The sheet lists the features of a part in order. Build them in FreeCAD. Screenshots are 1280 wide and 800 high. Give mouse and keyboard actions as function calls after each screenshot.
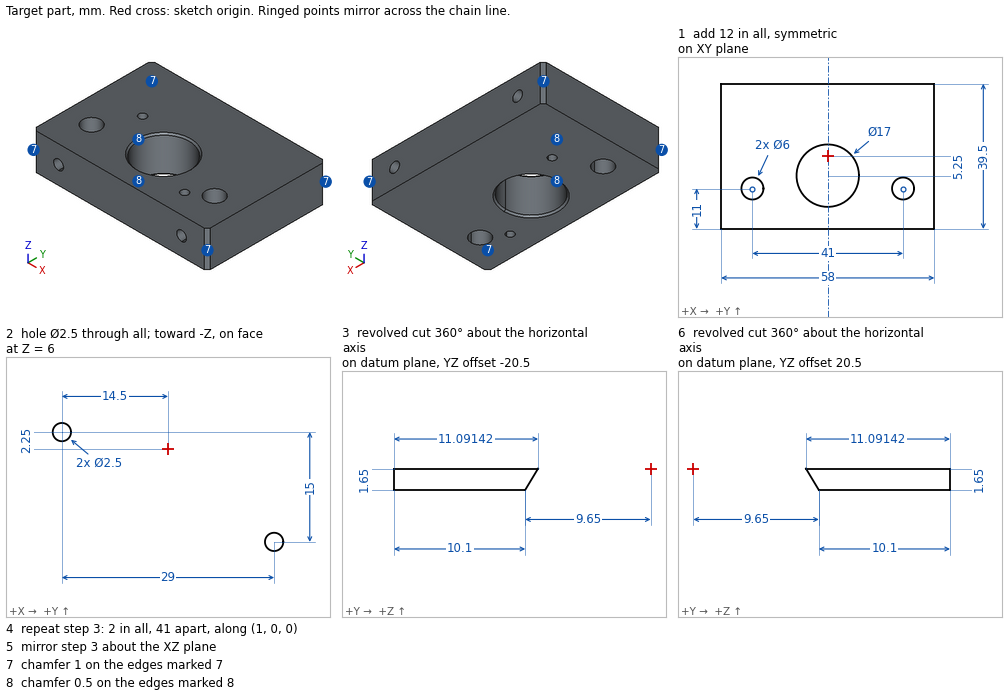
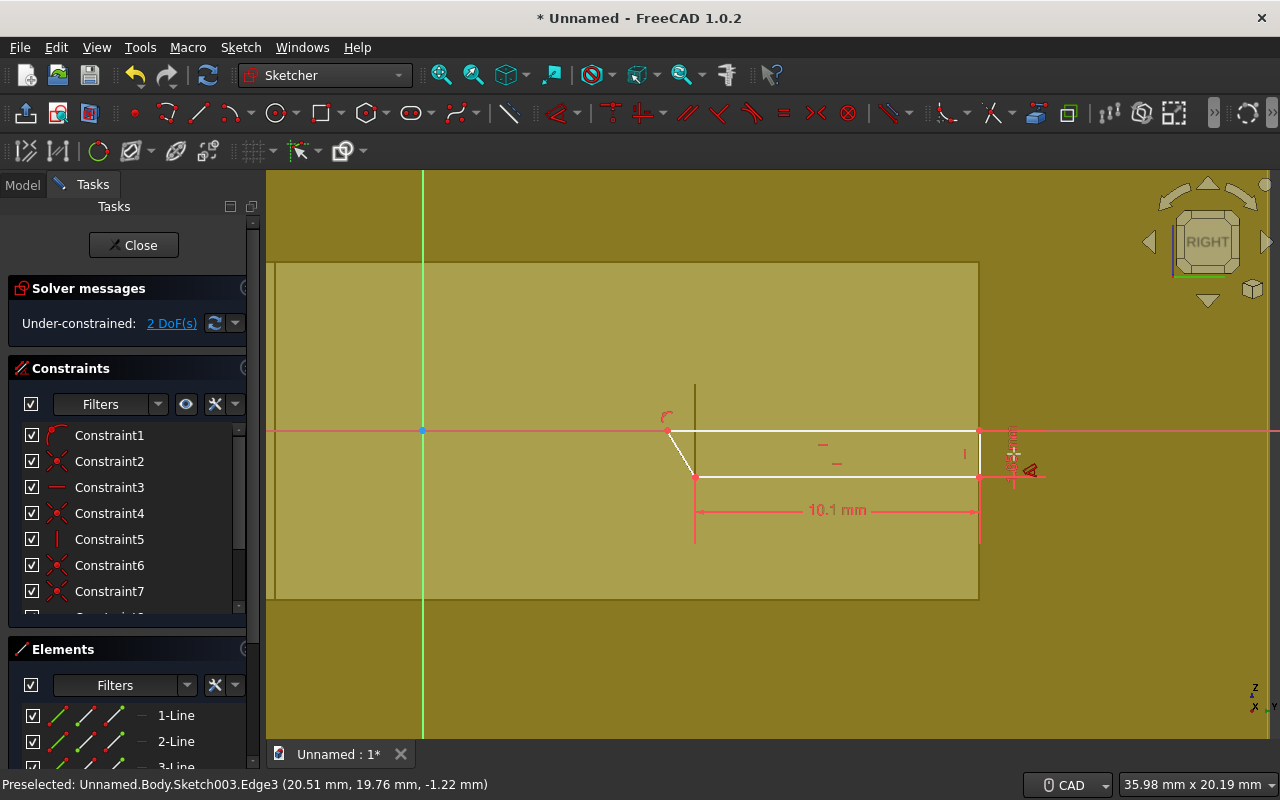
click(695, 477)
click(559, 511)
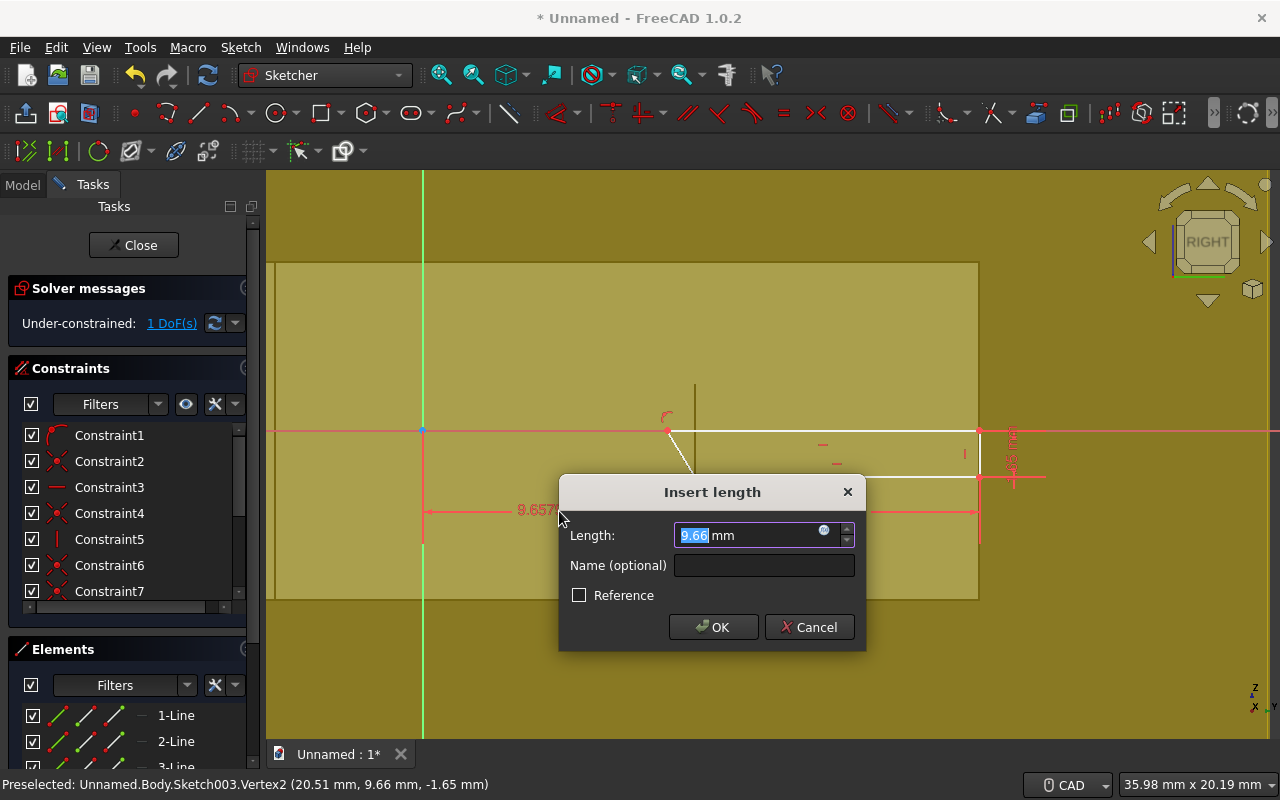
text(9.65)
key(Return)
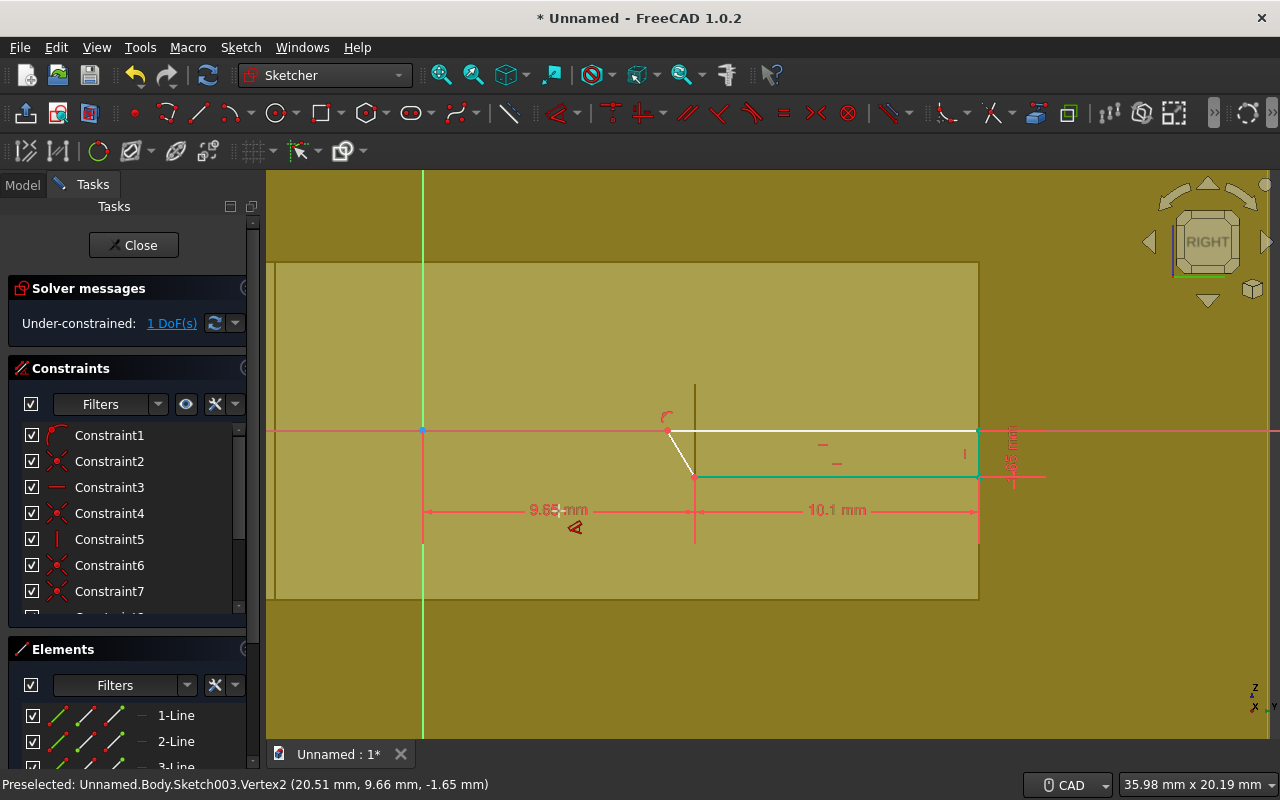
click(886, 431)
click(823, 397)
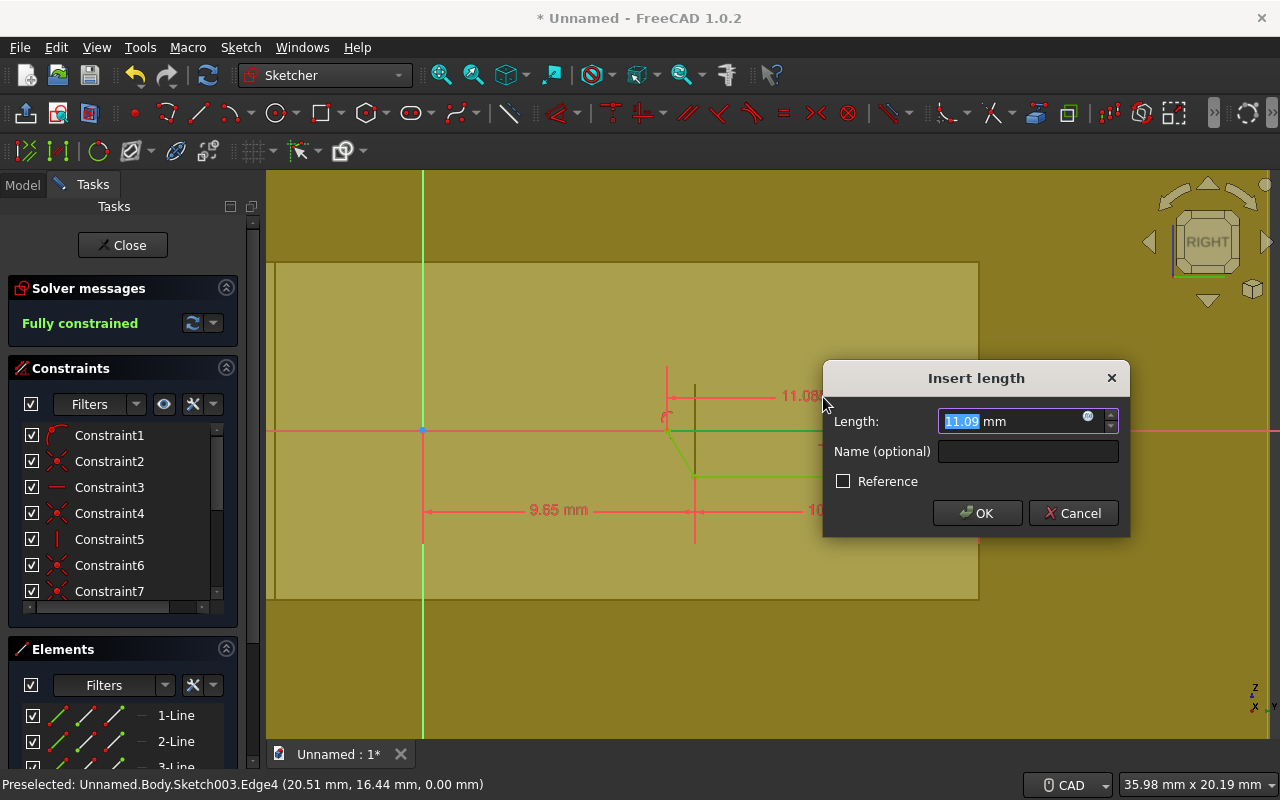
text(11.09142)
key(Return)
key(Escape)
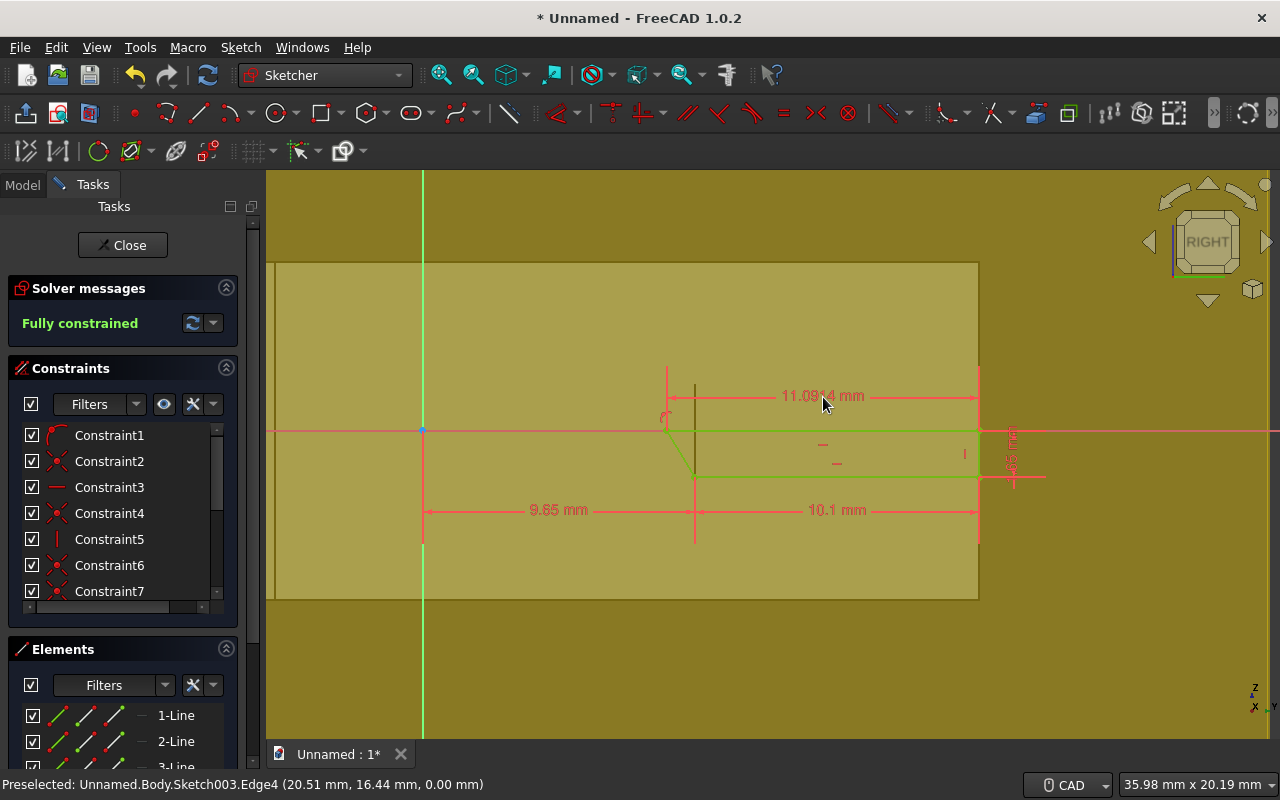
click(123, 245)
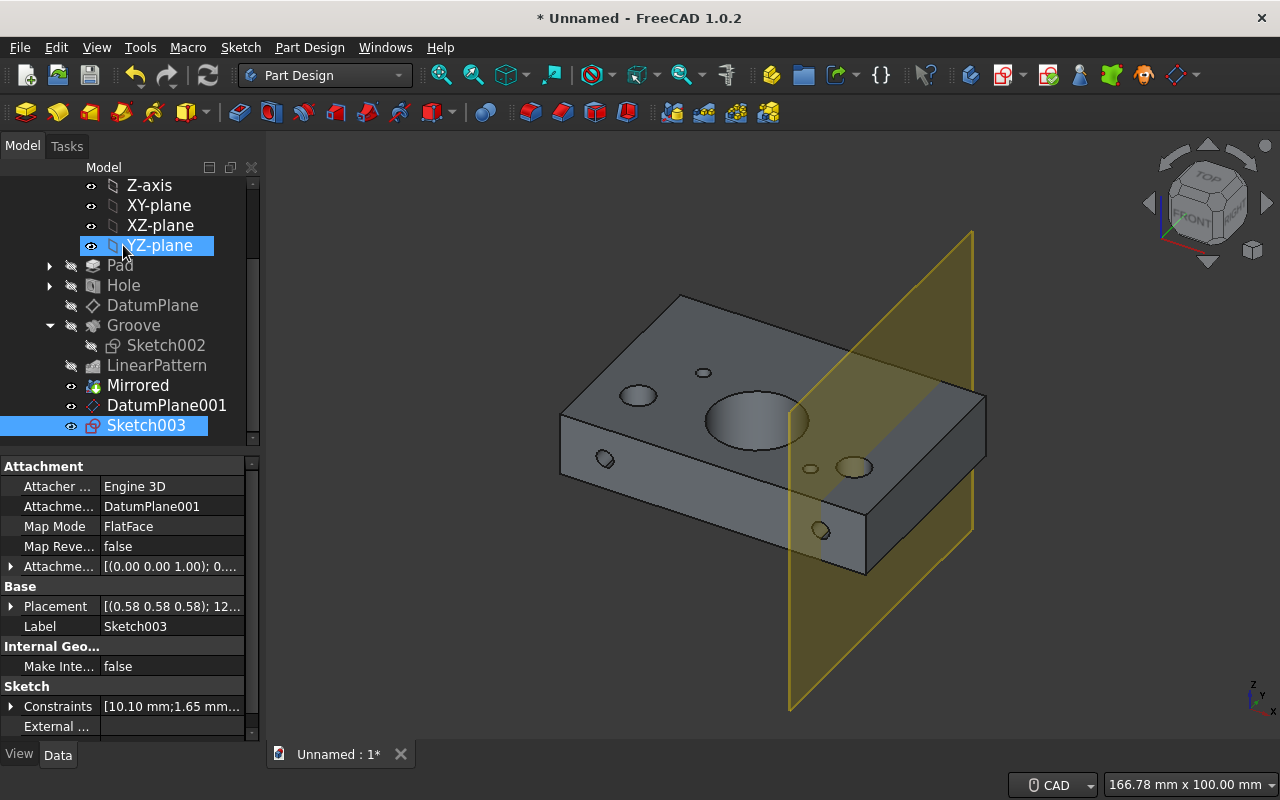
click(304, 112)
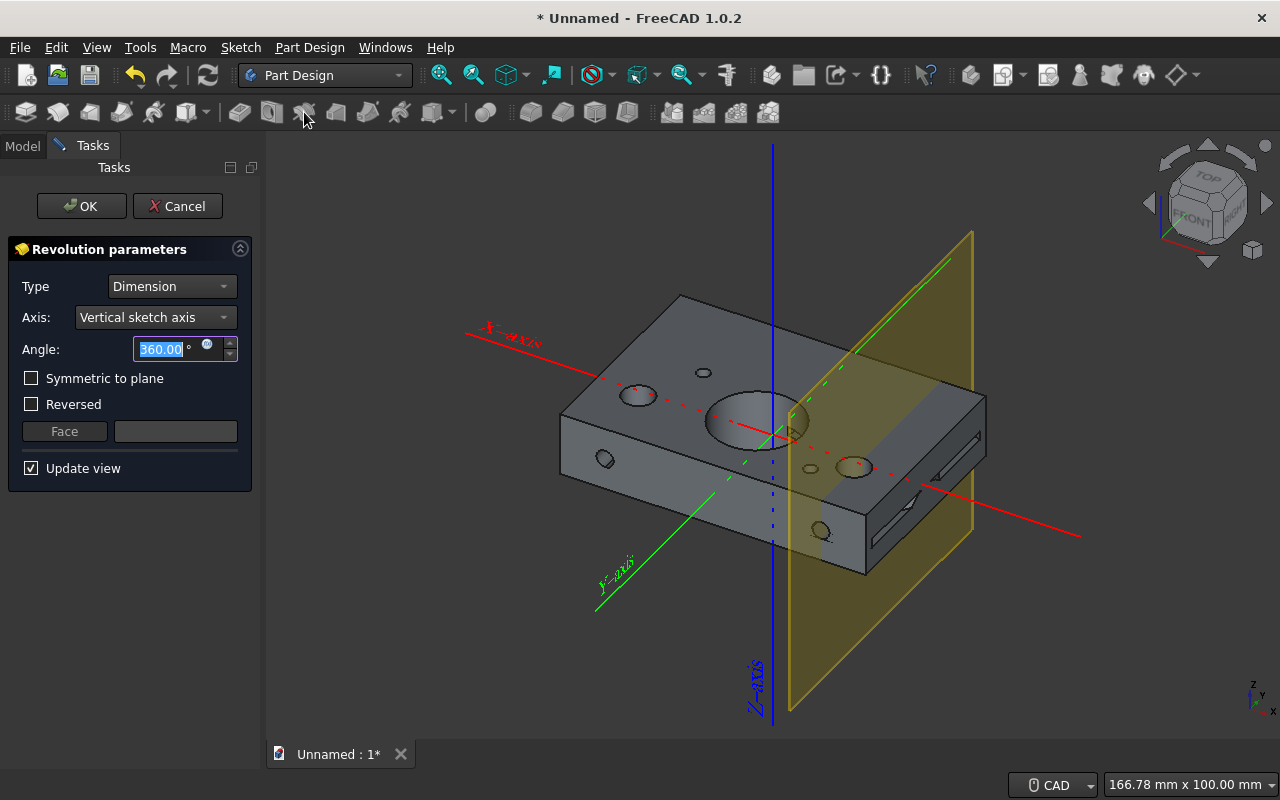
click(156, 318)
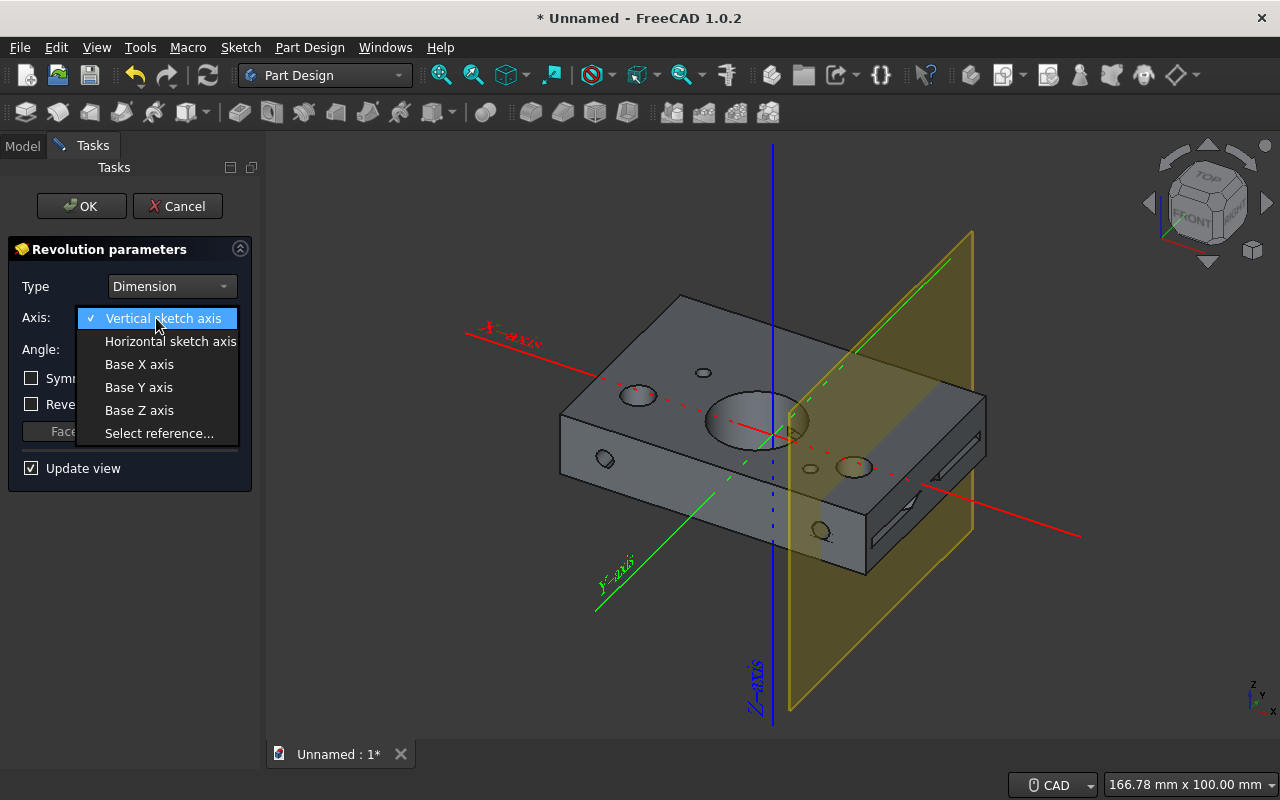
click(156, 342)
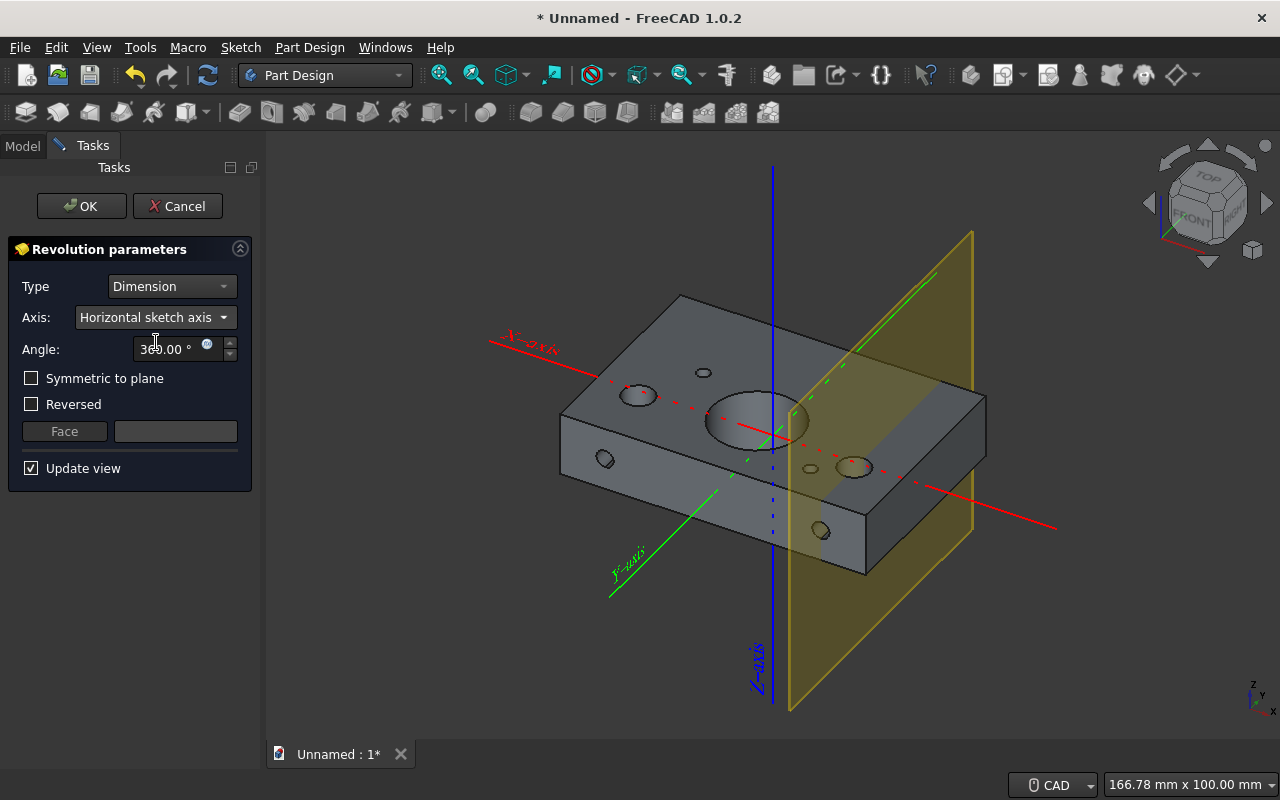
click(82, 206)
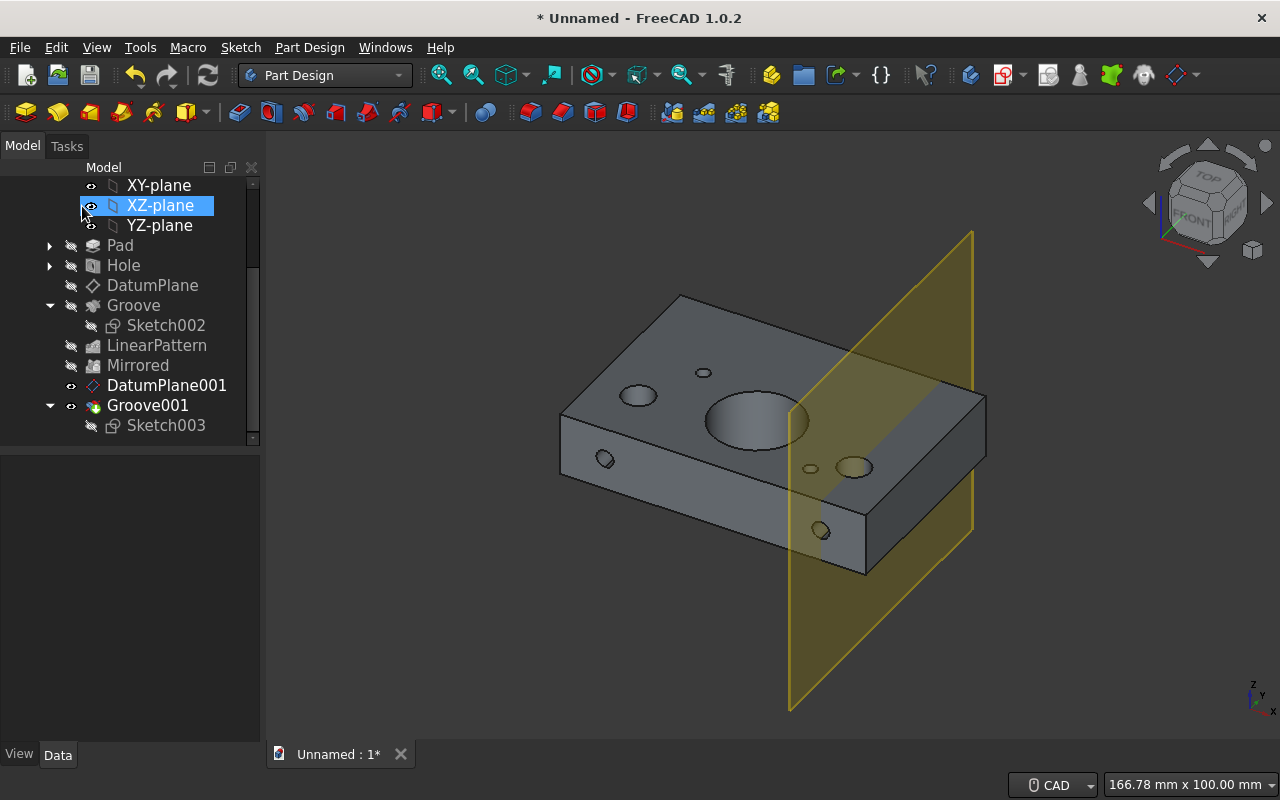
click(116, 386)
key(space)